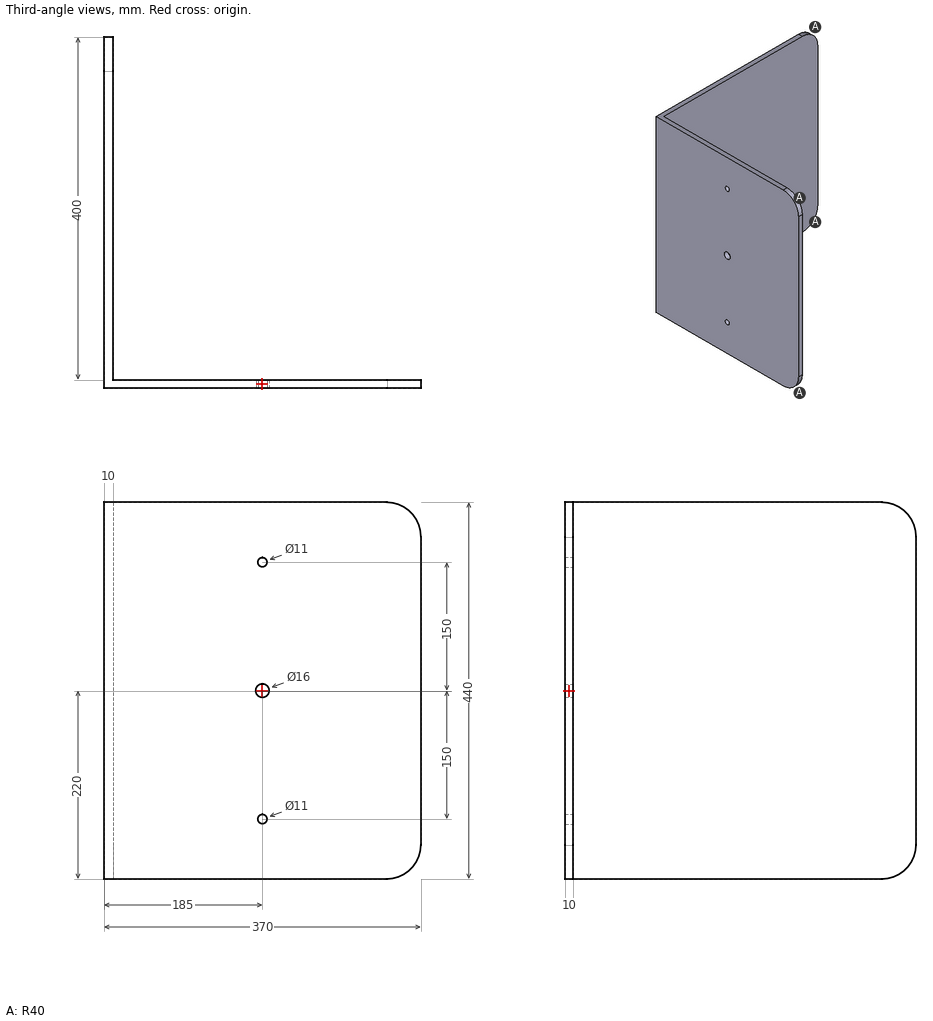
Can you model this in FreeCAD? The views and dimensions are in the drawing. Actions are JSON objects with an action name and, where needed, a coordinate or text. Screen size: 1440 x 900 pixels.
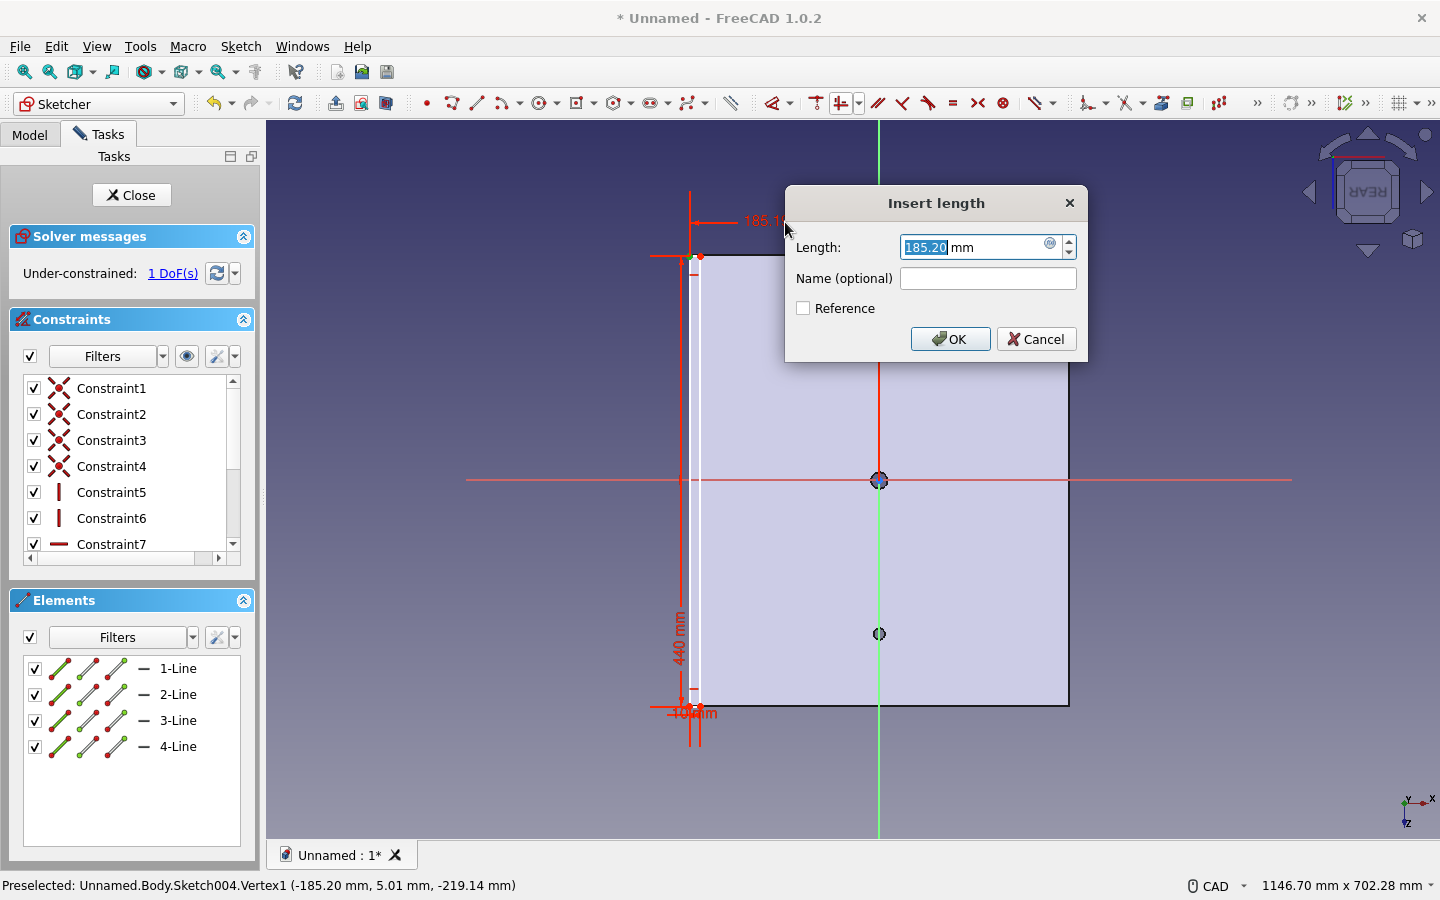
{"action": "type", "text": "185"}
{"action": "key", "text": "Return"}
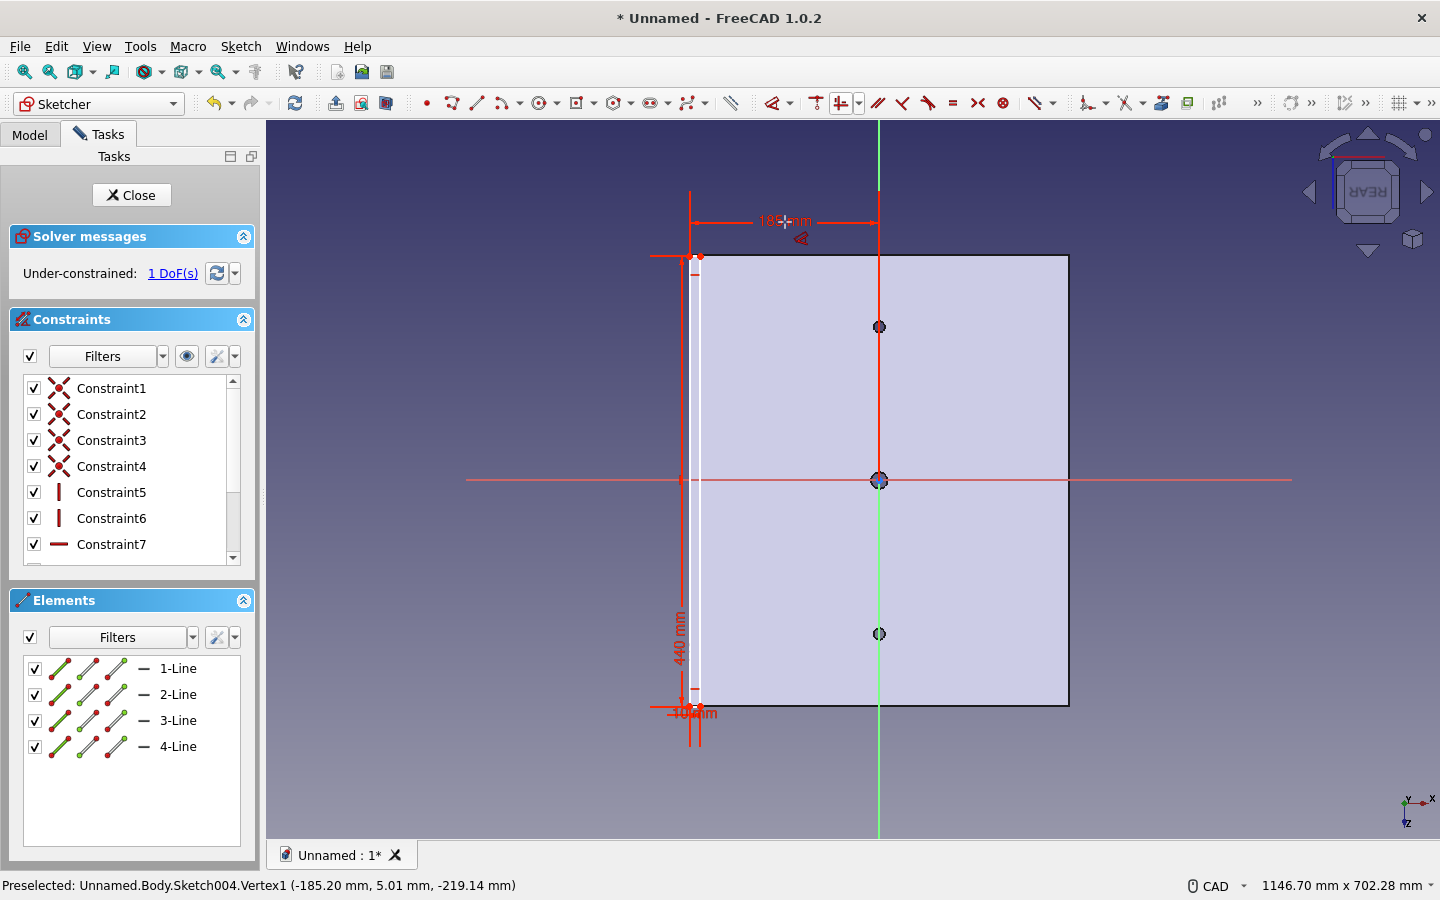
{"action": "left_click", "coordinate": [690, 256]}
{"action": "left_click", "coordinate": [913, 368]}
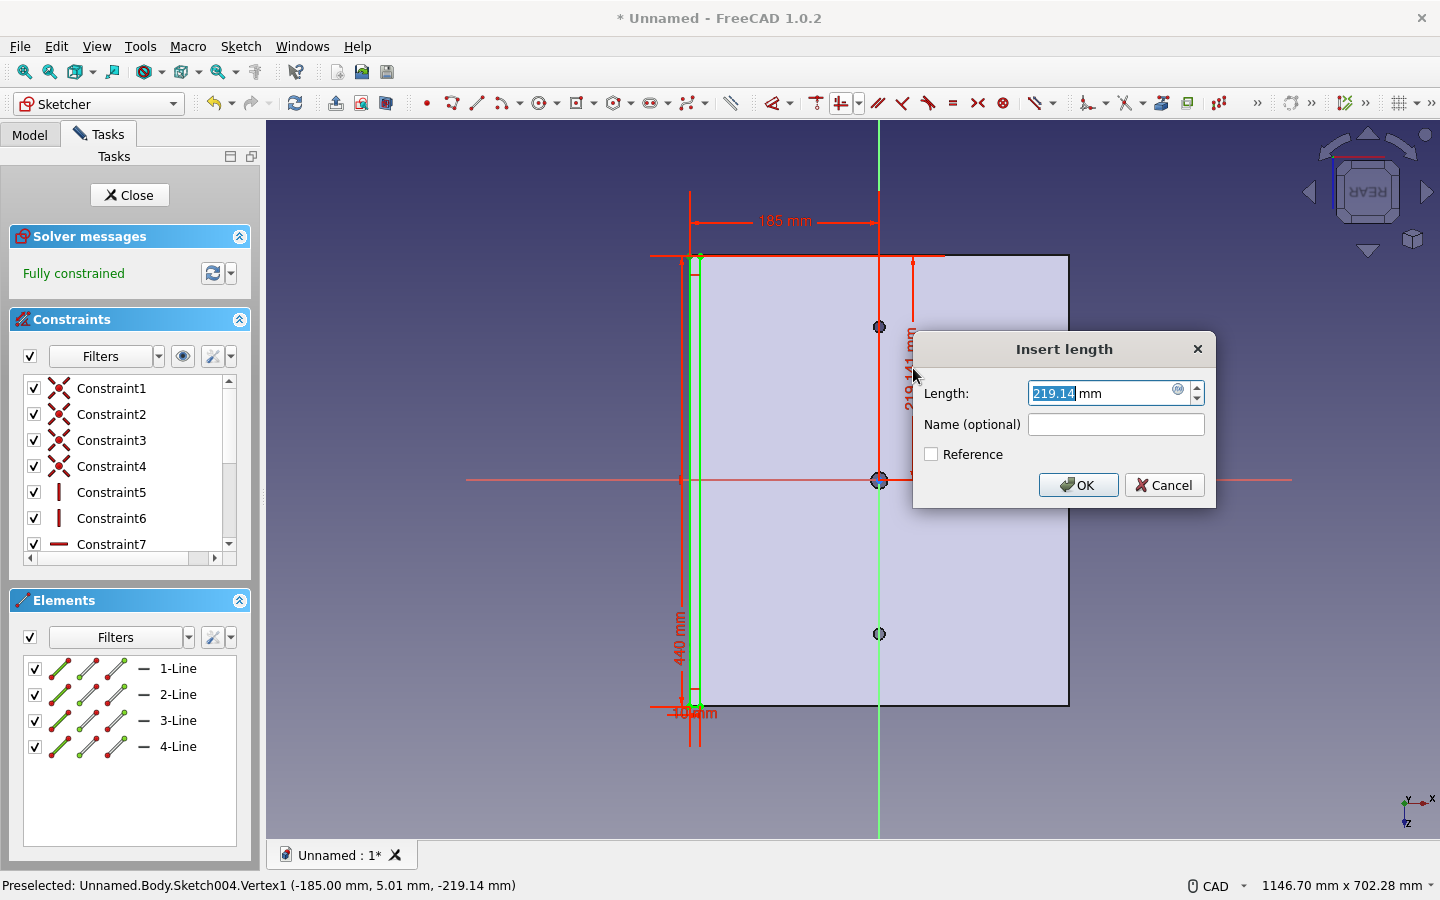
{"action": "type", "text": "220"}
{"action": "key", "text": "Return"}
{"action": "key", "text": "Escape"}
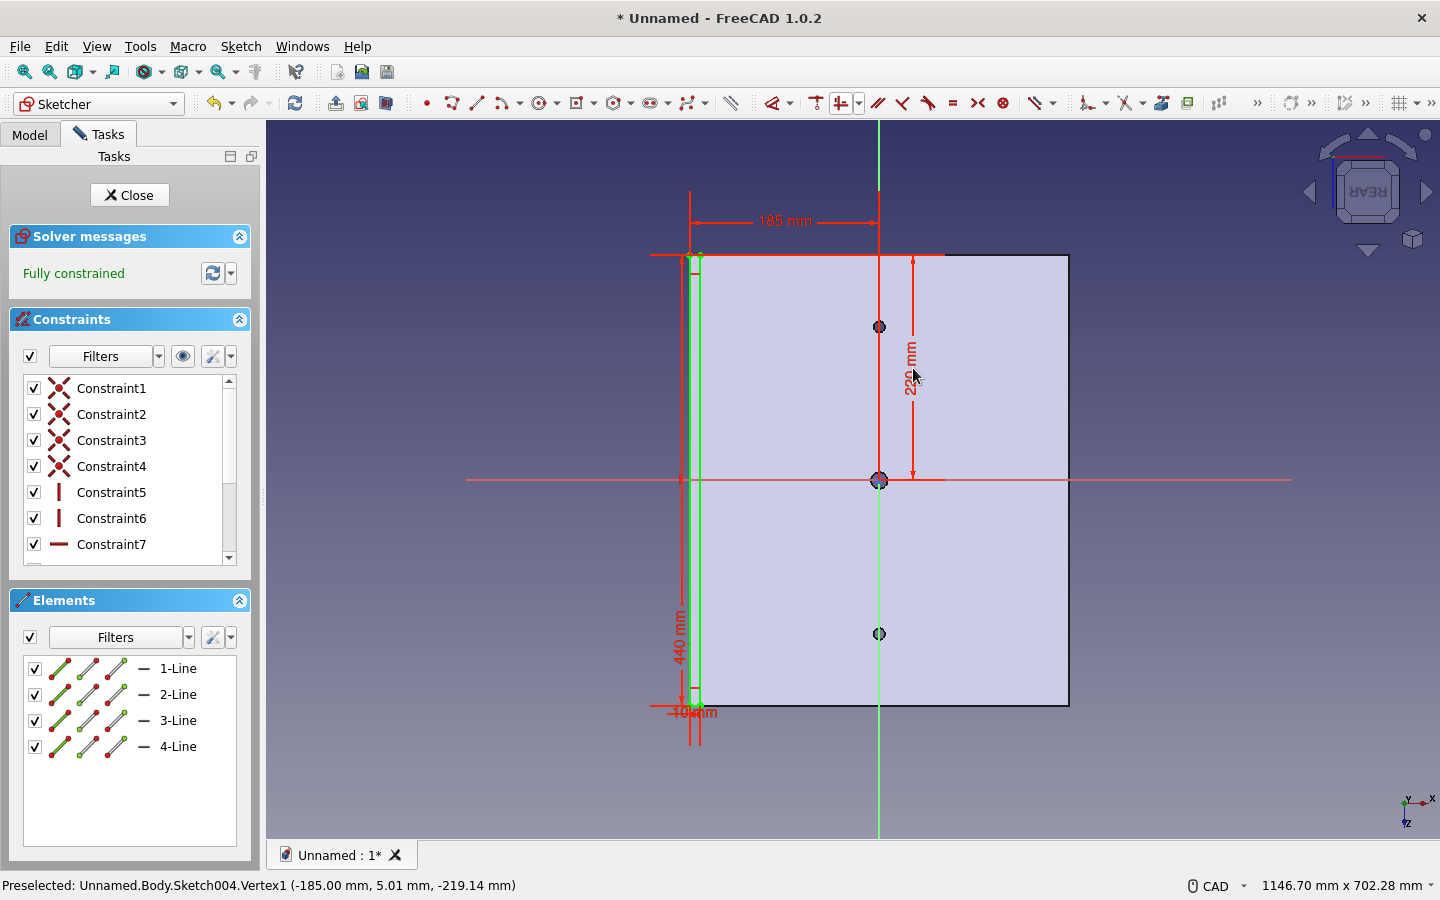
{"action": "left_click", "coordinate": [130, 195]}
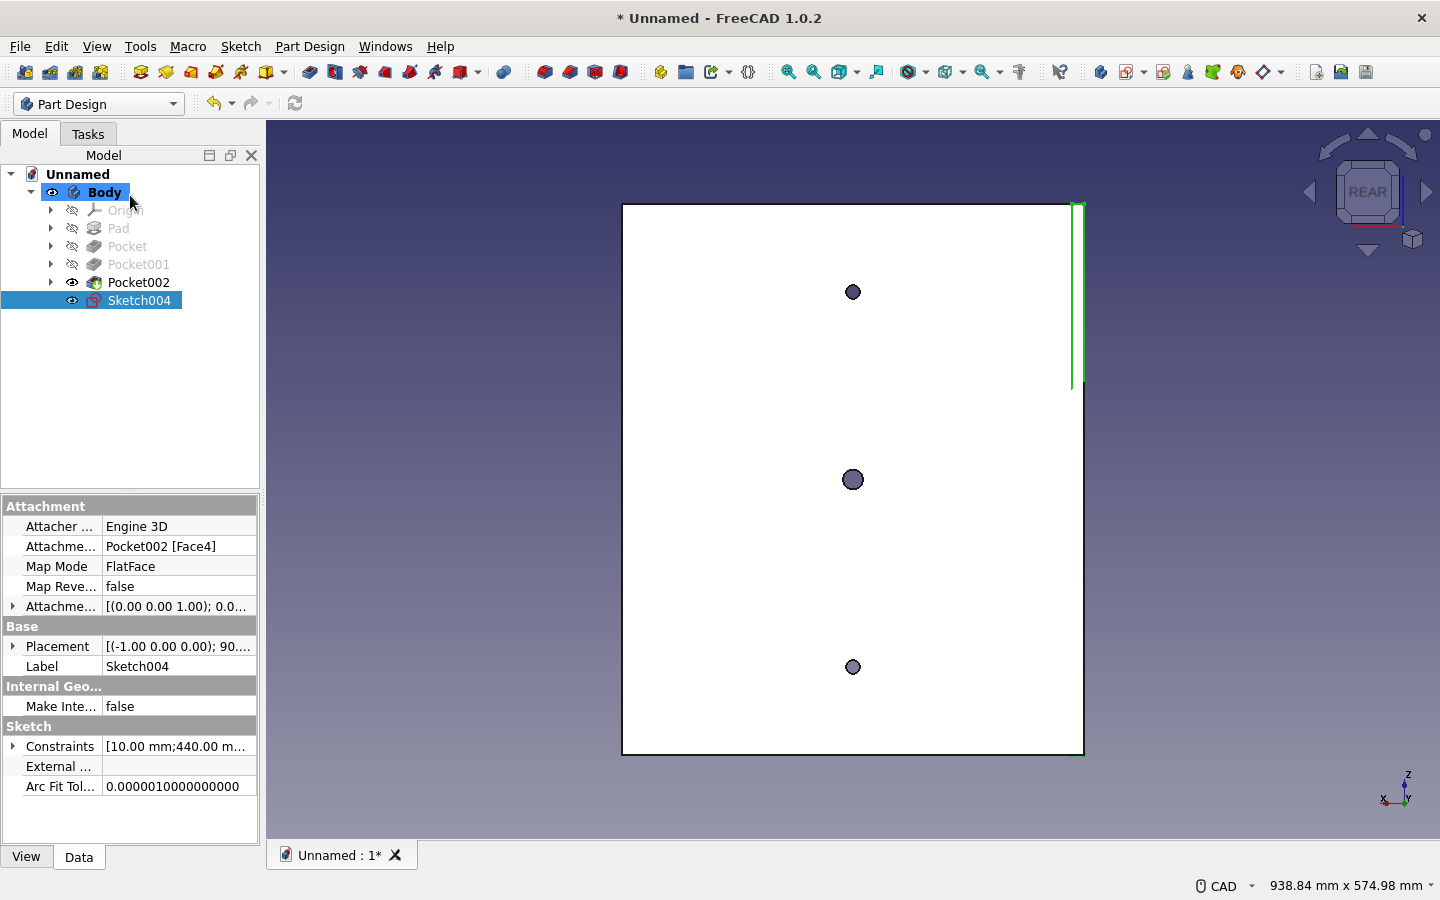
{"action": "left_click", "coordinate": [141, 72]}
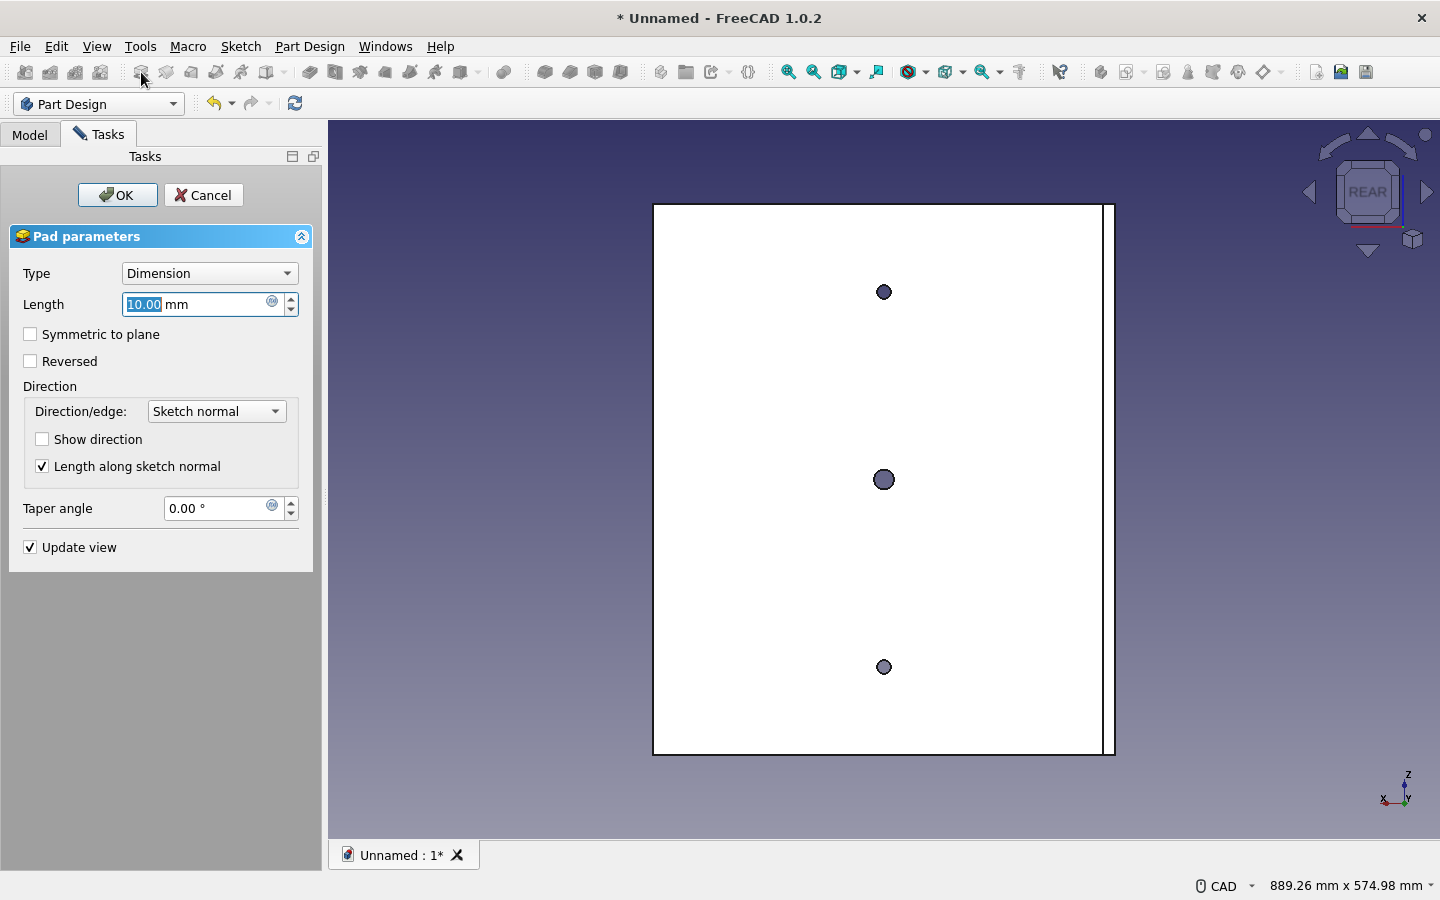
{"action": "type", "text": "400"}
{"action": "key", "text": "Tab"}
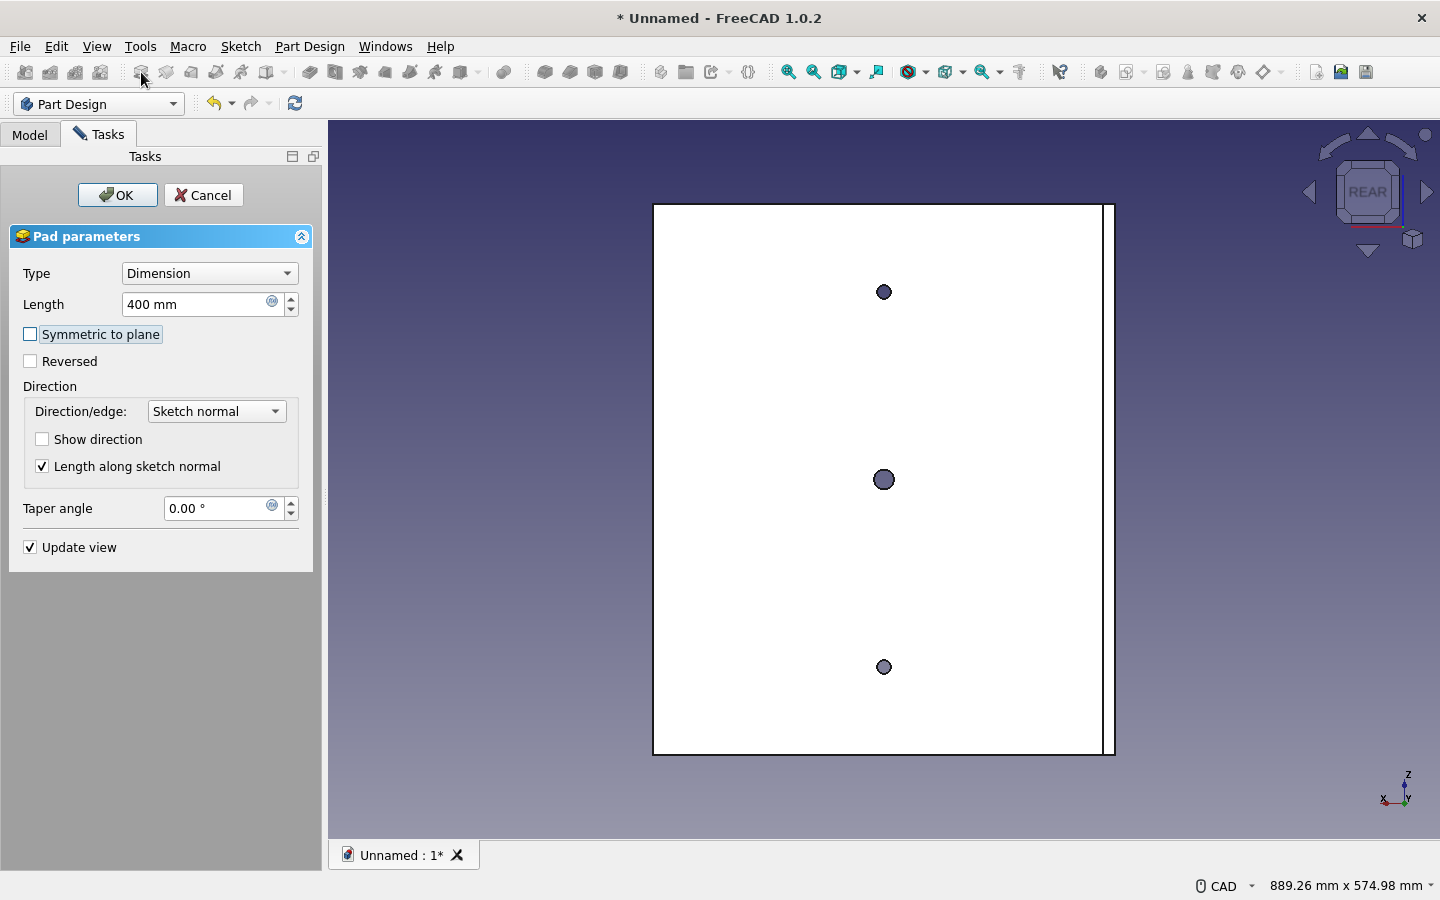
{"action": "left_click", "coordinate": [118, 195]}